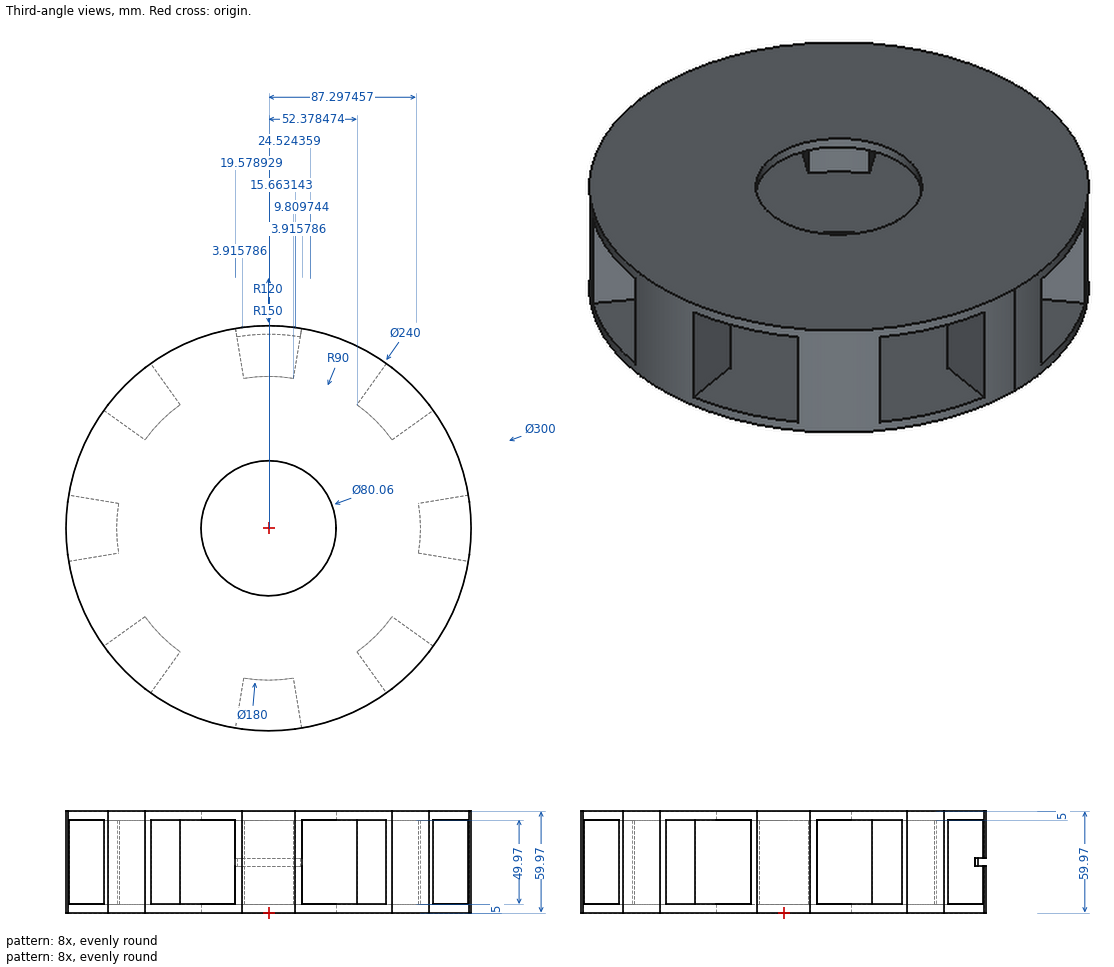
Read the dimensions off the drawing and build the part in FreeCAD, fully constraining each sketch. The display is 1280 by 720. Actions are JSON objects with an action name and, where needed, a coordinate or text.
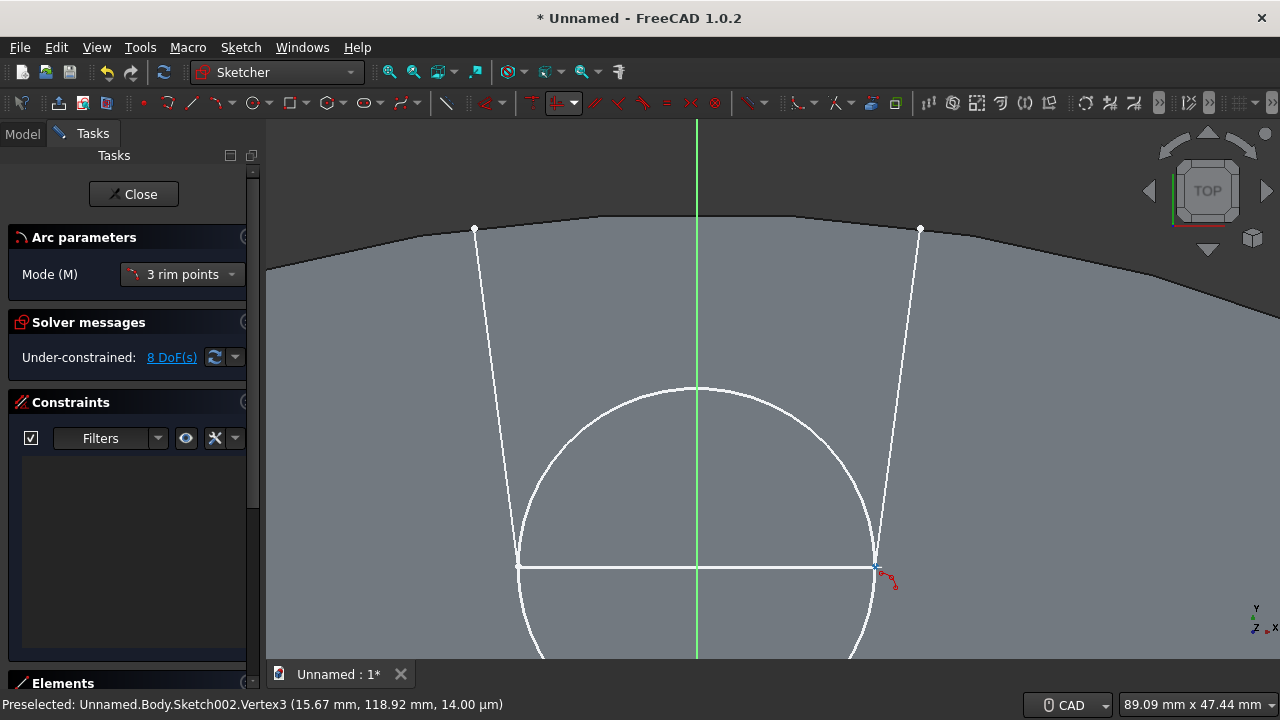
{"action": "scroll", "coordinate": [732, 555], "scroll_direction": "up", "scroll_amount": 2}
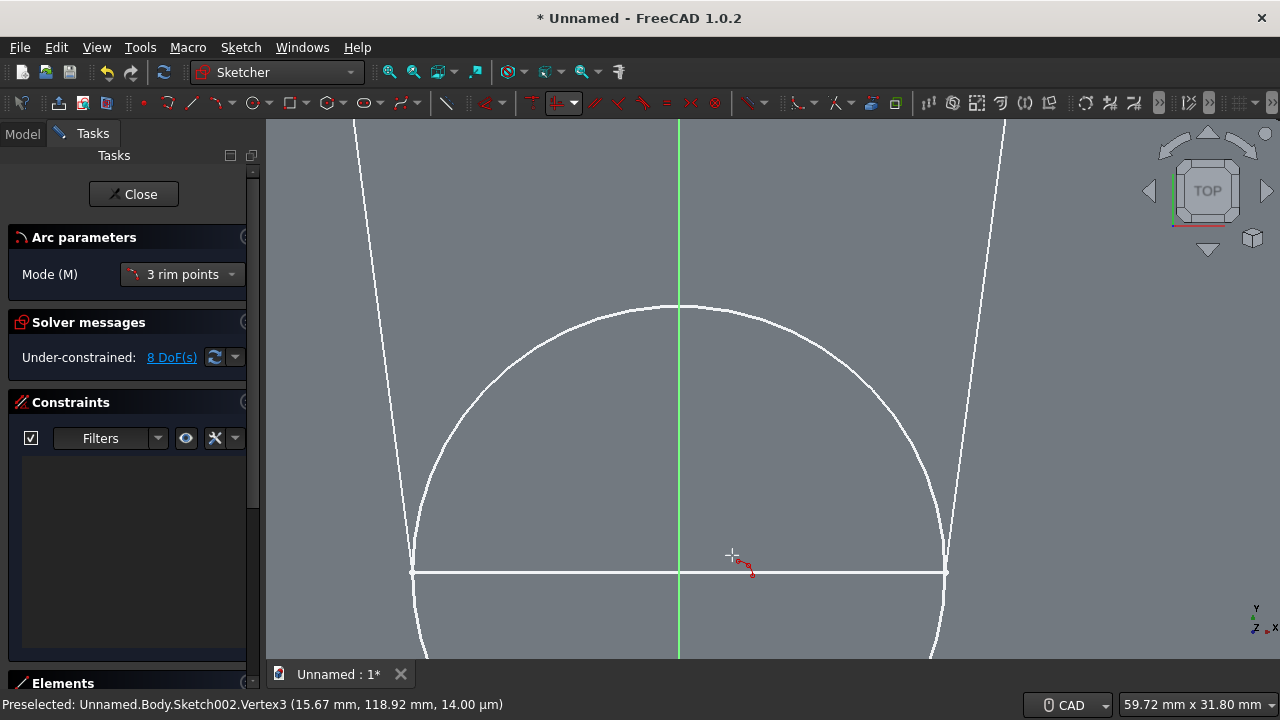
{"action": "left_click", "coordinate": [732, 555]}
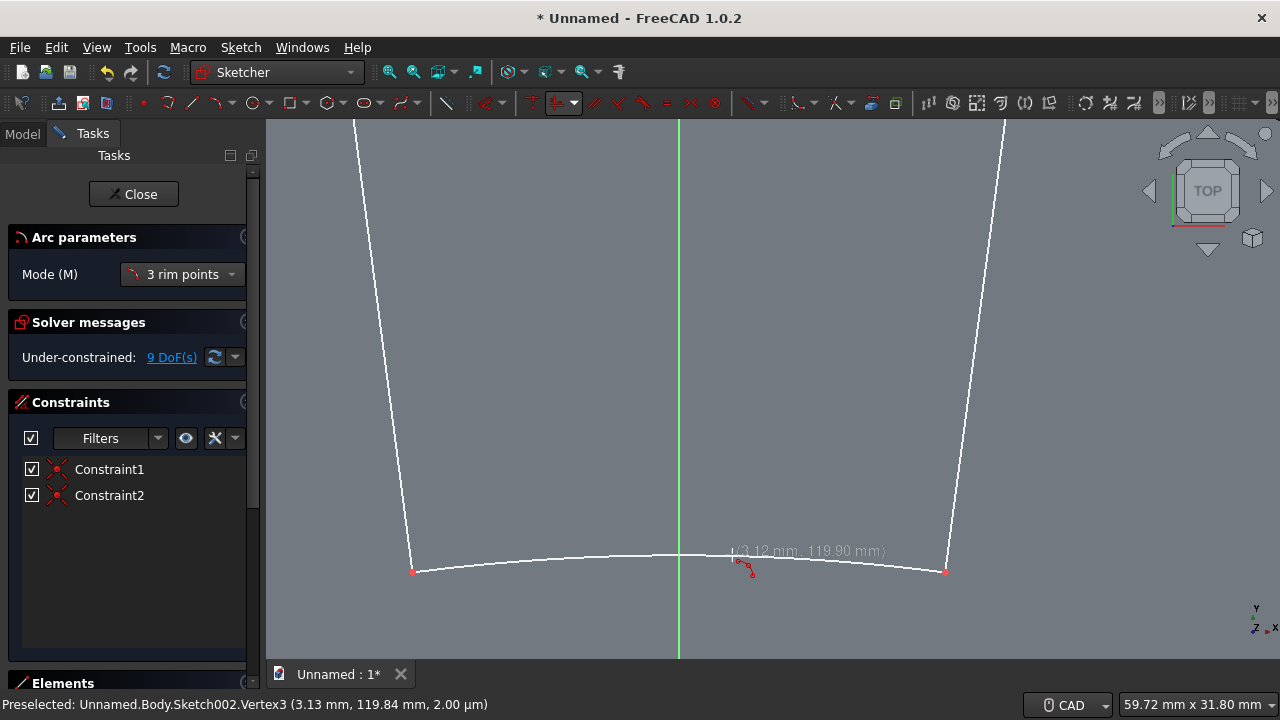
{"action": "scroll", "coordinate": [756, 553], "scroll_direction": "down", "scroll_amount": 2}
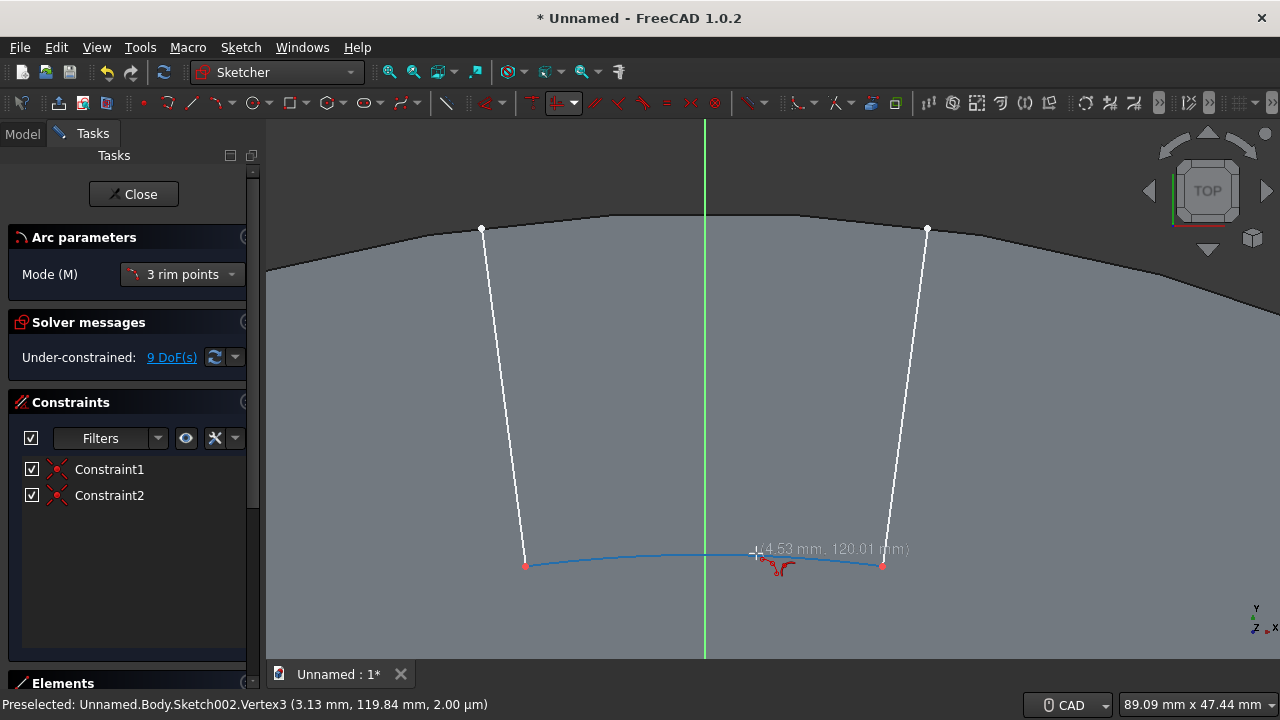
{"action": "left_click", "coordinate": [928, 228]}
{"action": "left_click", "coordinate": [482, 228]}
{"action": "left_click", "coordinate": [749, 213]}
{"action": "key", "text": "Escape"}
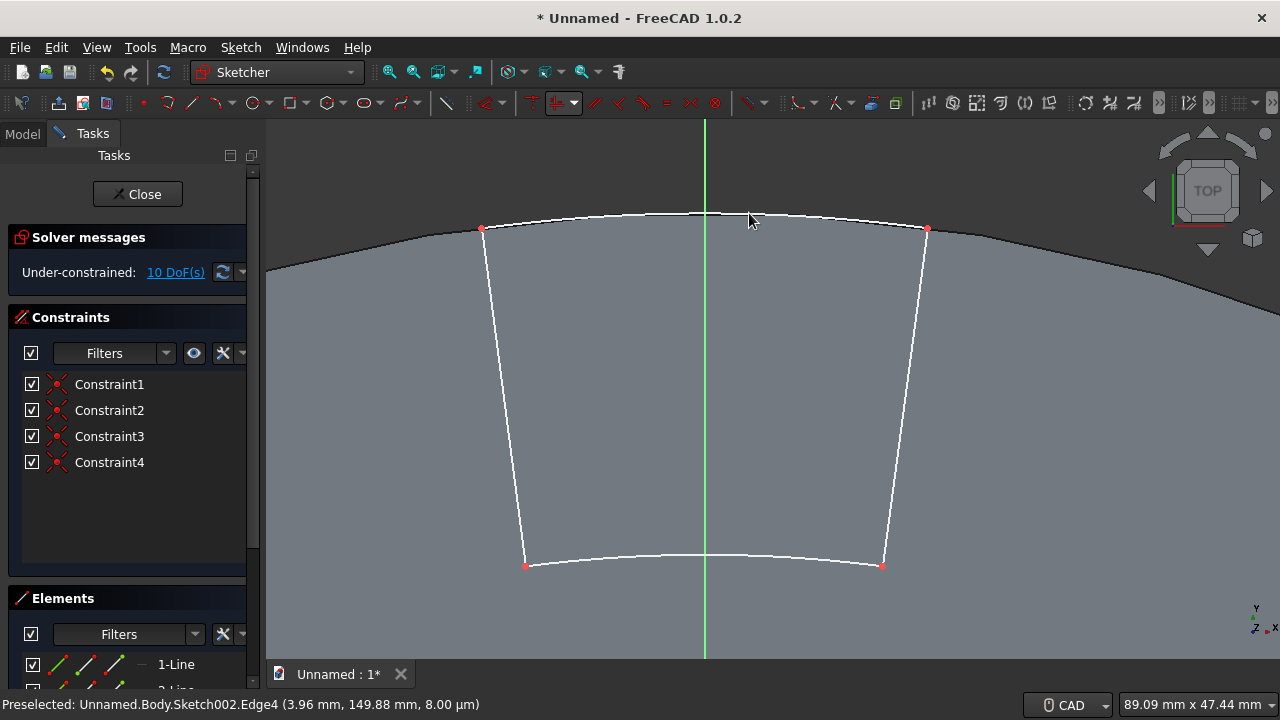
{"action": "left_click", "coordinate": [776, 557]}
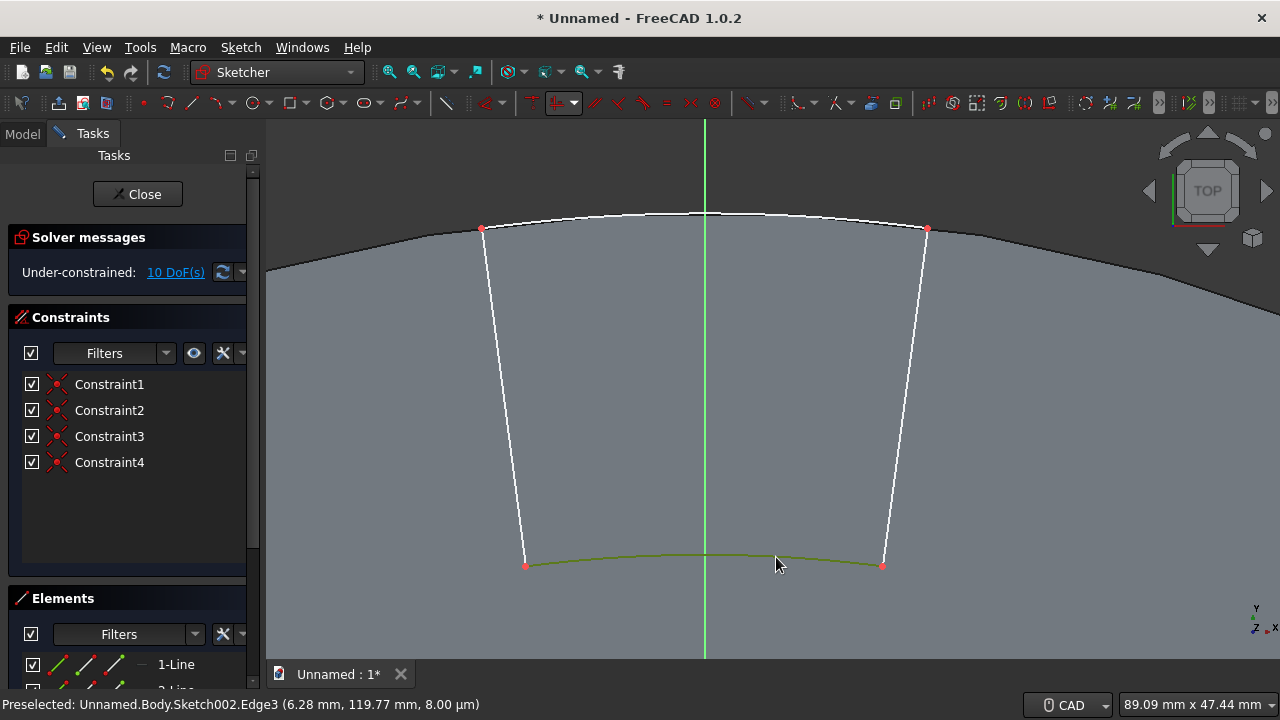
{"action": "left_click", "coordinate": [794, 216]}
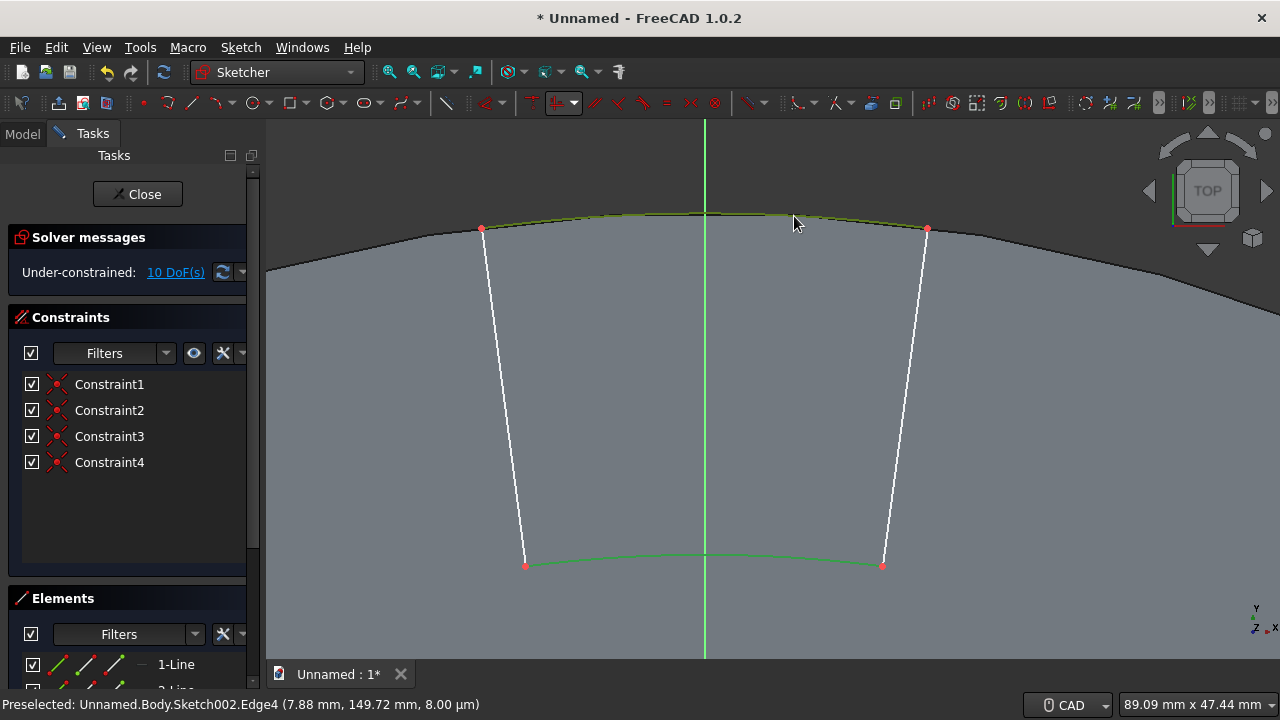
{"action": "left_click", "coordinate": [532, 104]}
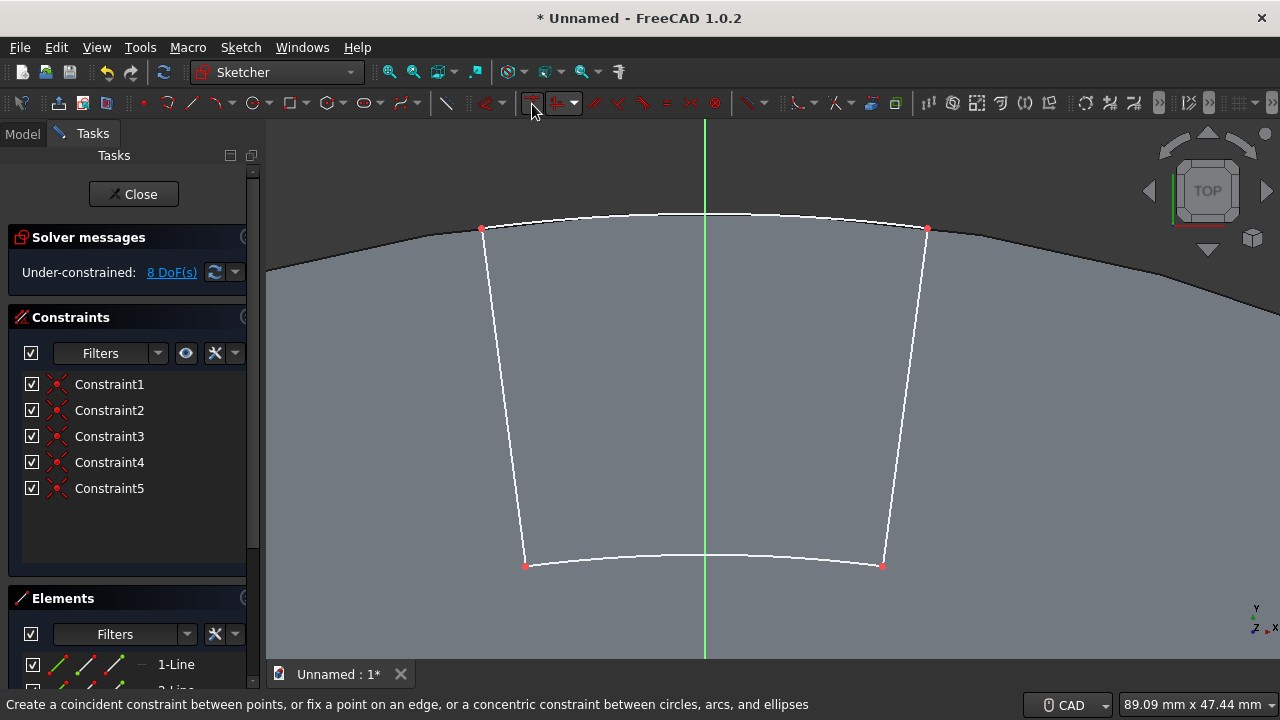
{"action": "scroll", "coordinate": [704, 216], "scroll_direction": "down", "scroll_amount": 8}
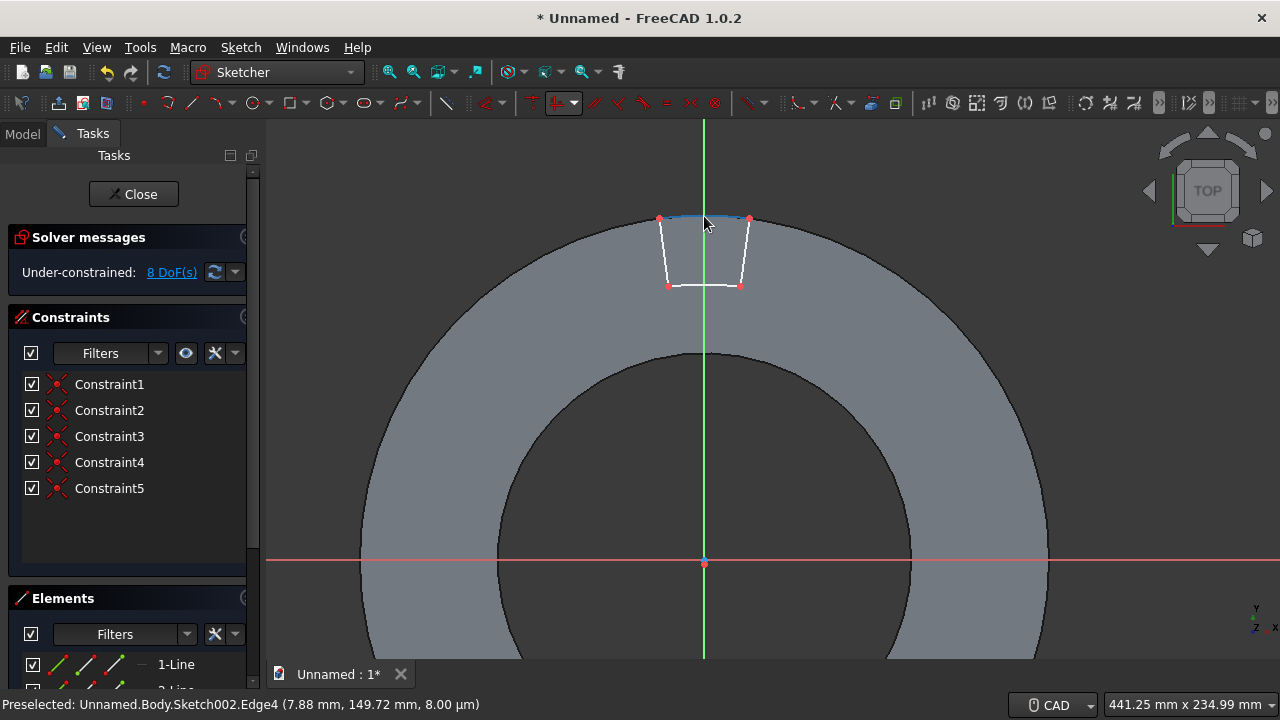
{"action": "left_click_drag", "start_coordinate": [694, 550], "coordinate": [714, 575]}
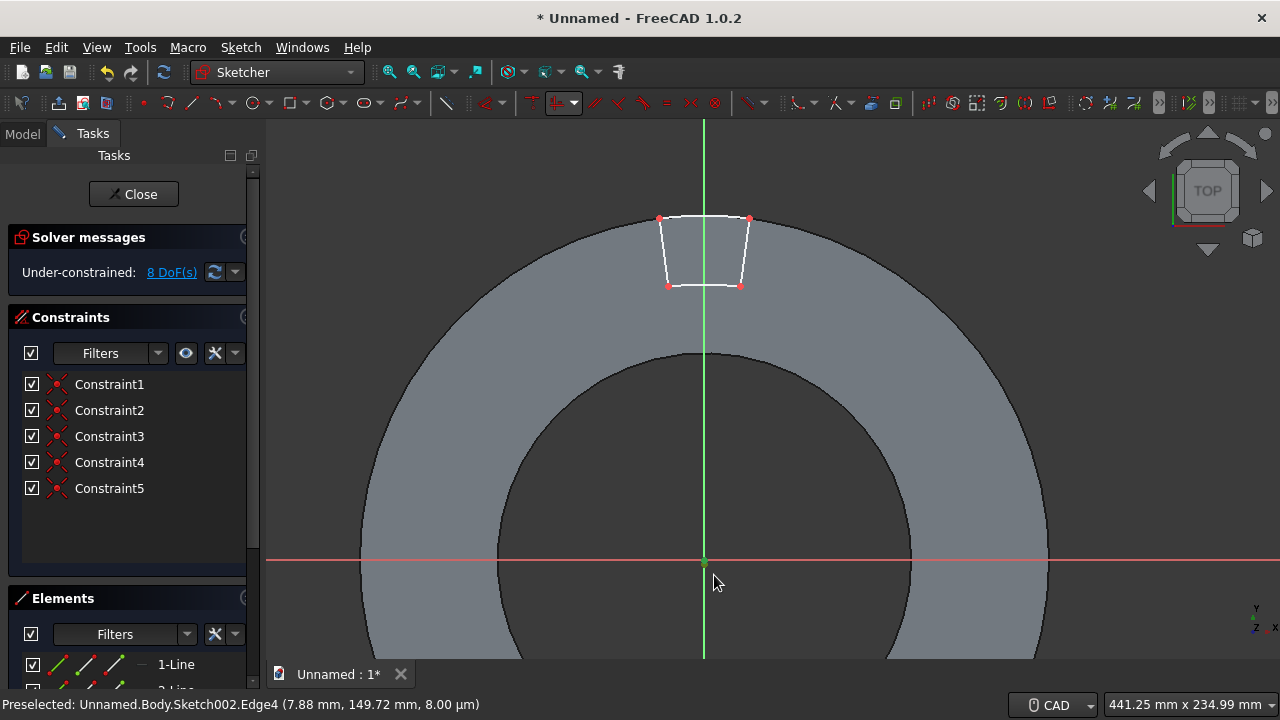
{"action": "key", "text": "c"}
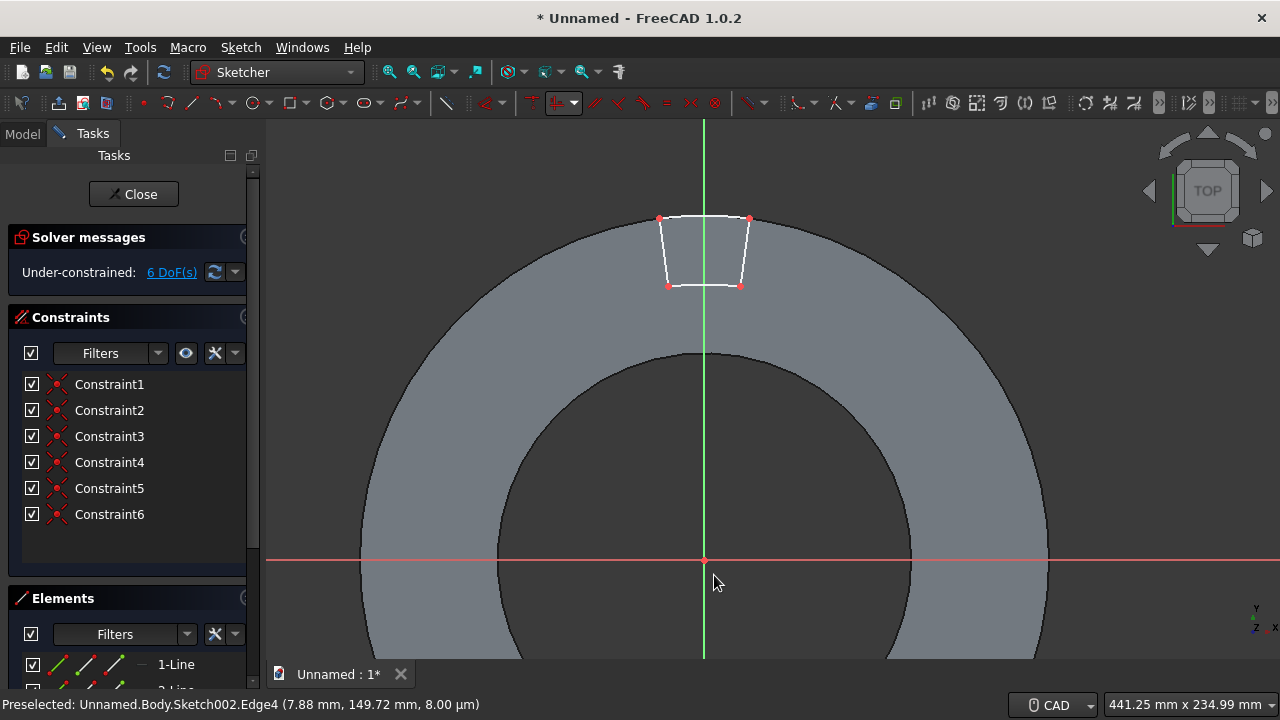
{"action": "left_click", "coordinate": [486, 104]}